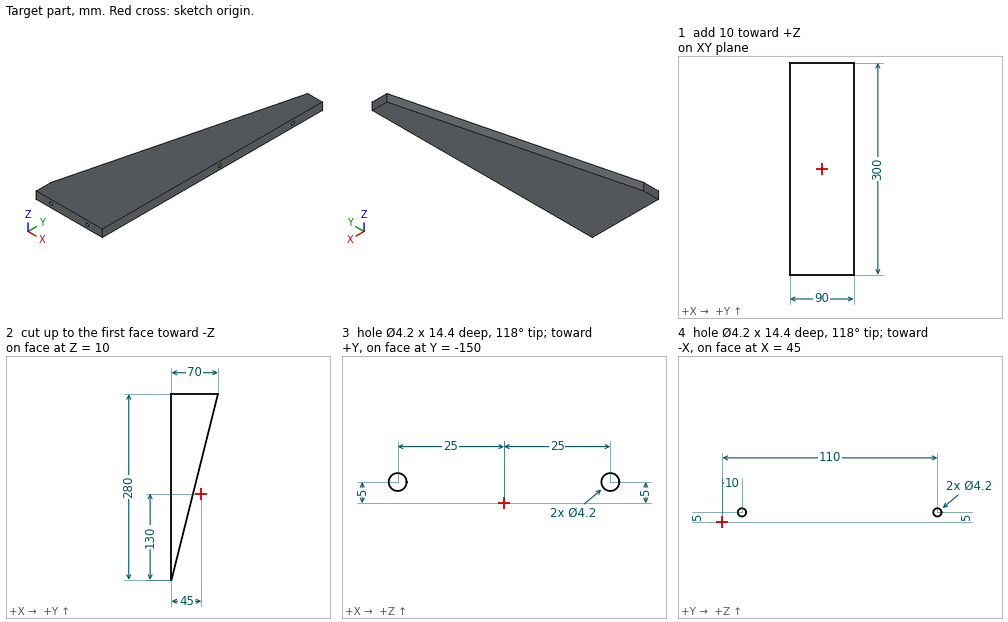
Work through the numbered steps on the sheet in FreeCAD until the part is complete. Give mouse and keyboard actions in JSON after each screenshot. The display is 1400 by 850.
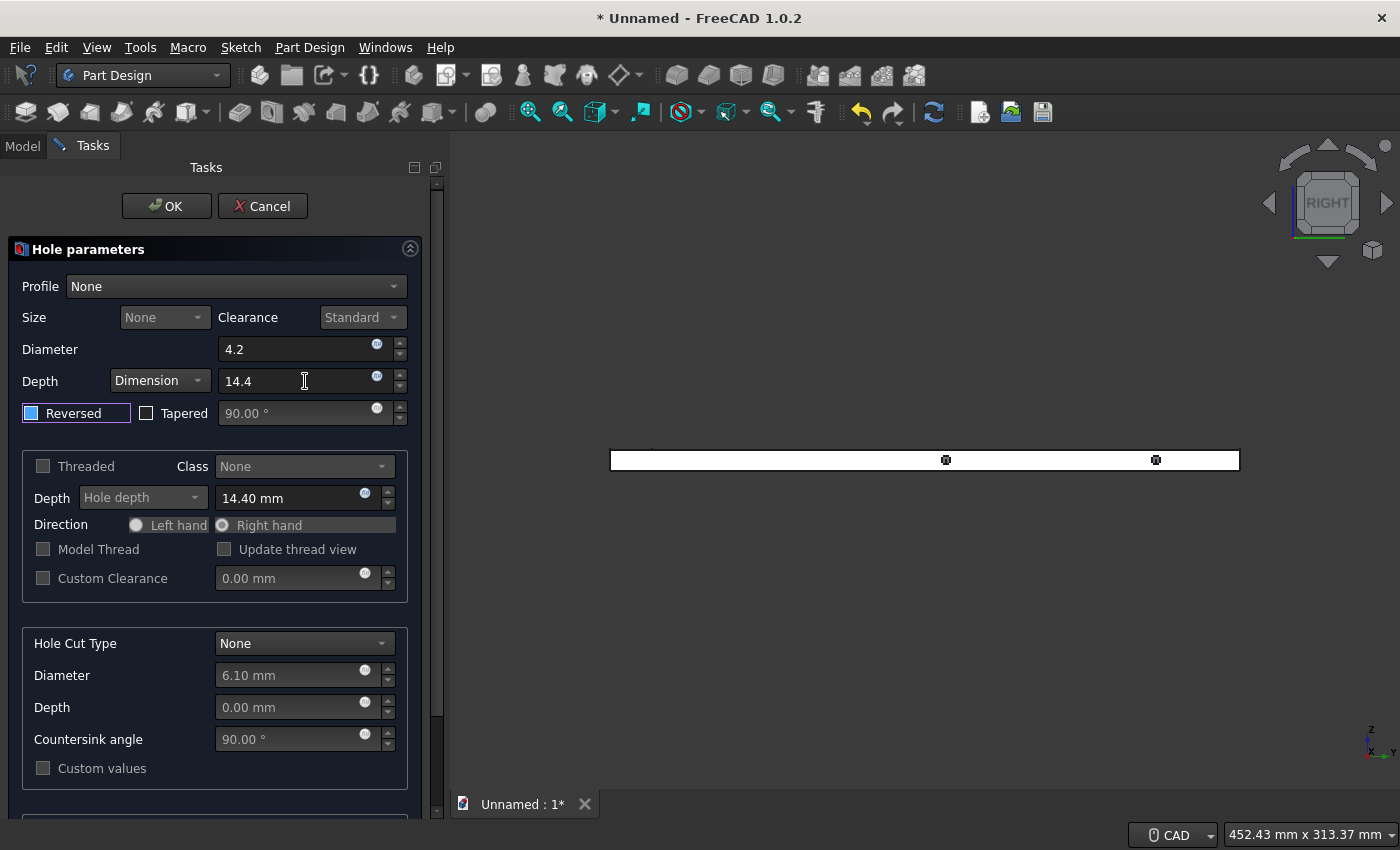
{"action": "left_click", "coordinate": [167, 206]}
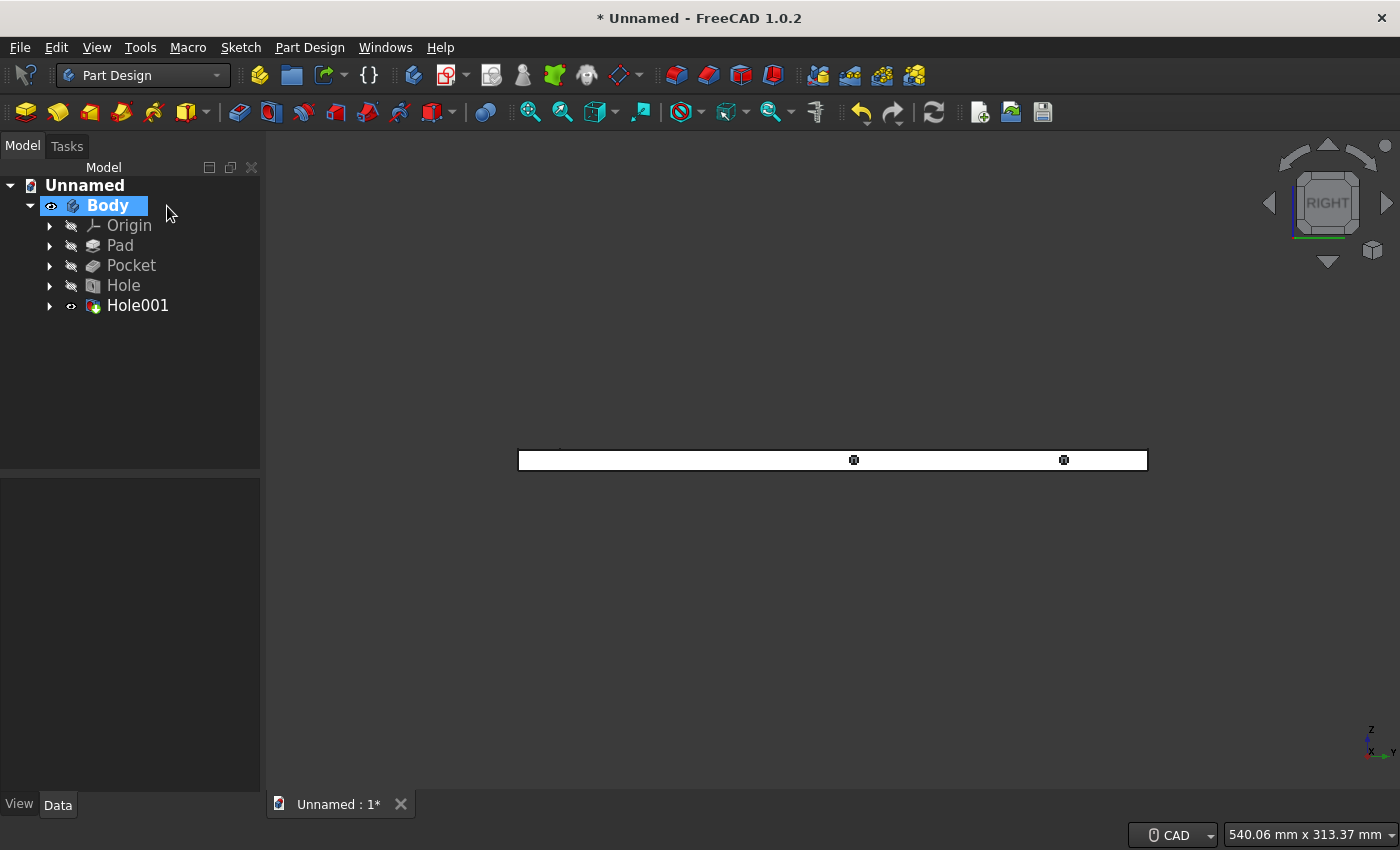
{"action": "key", "text": "0"}